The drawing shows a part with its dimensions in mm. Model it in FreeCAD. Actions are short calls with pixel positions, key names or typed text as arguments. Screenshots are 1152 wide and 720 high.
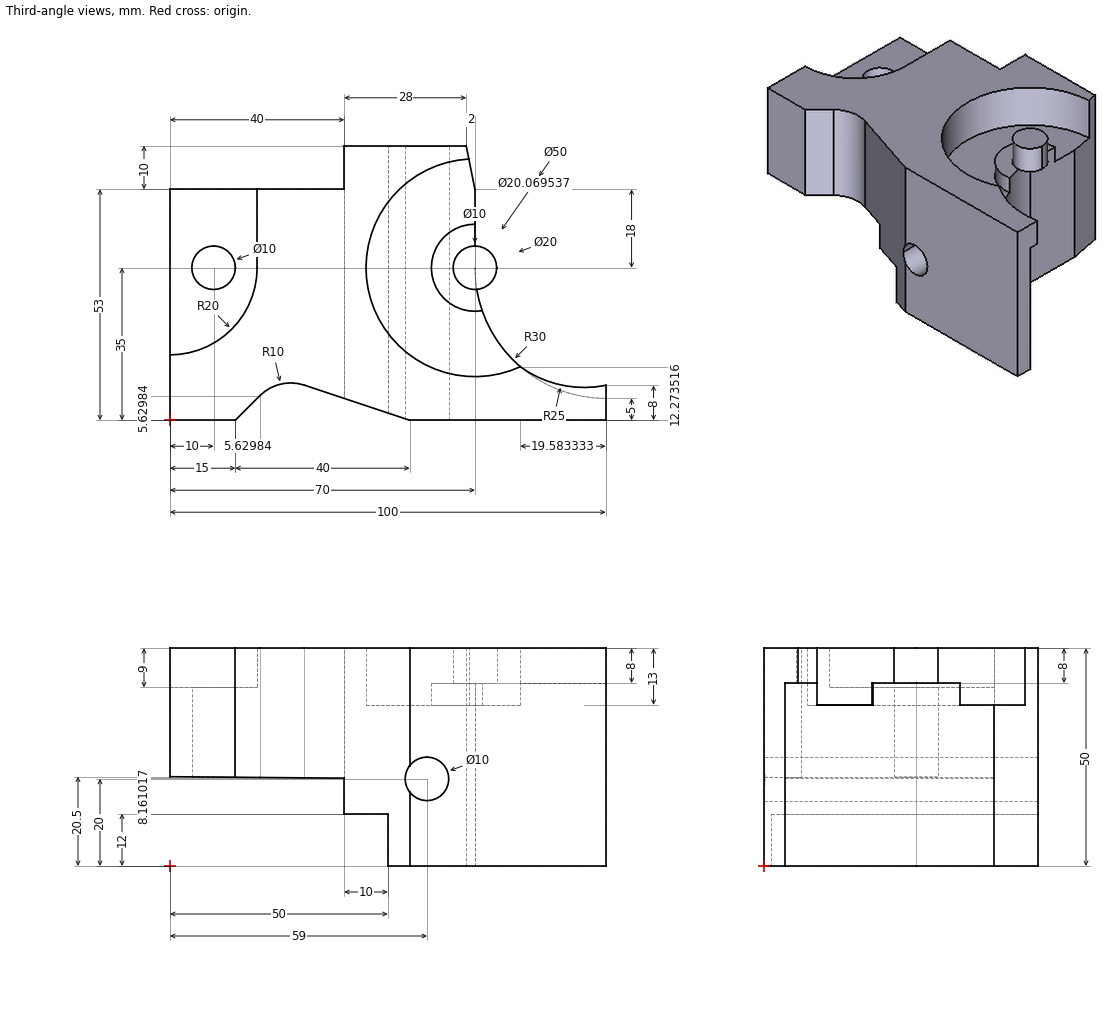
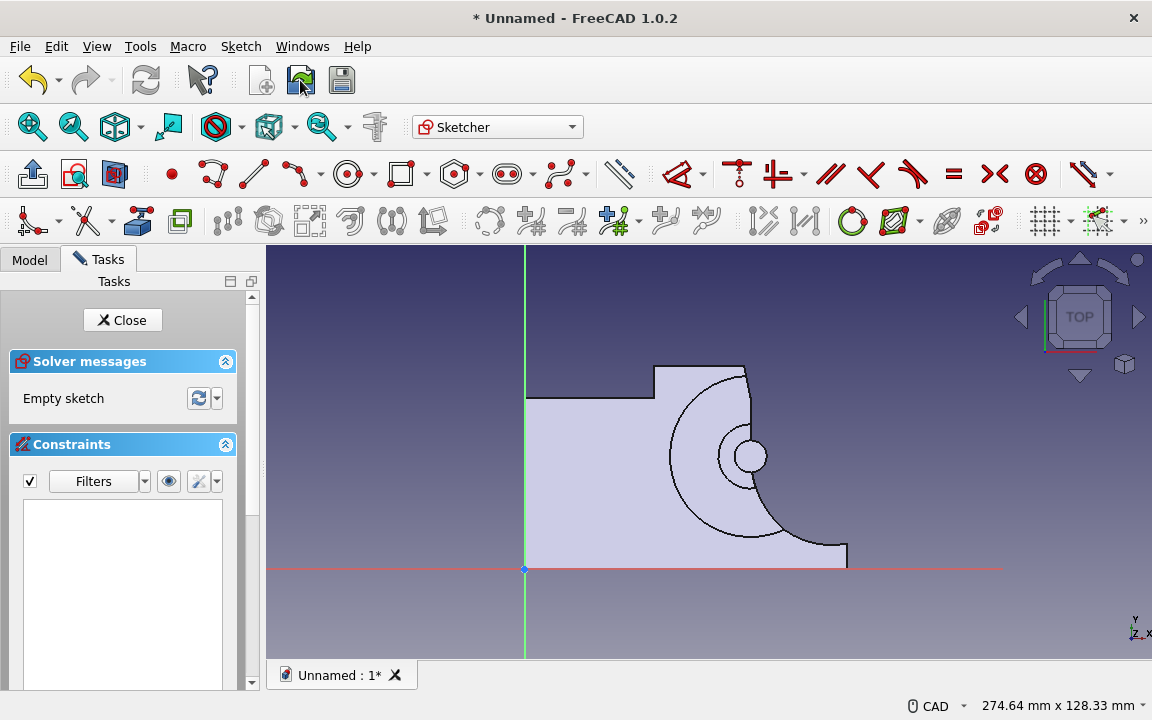
scroll(598, 616, up, 5)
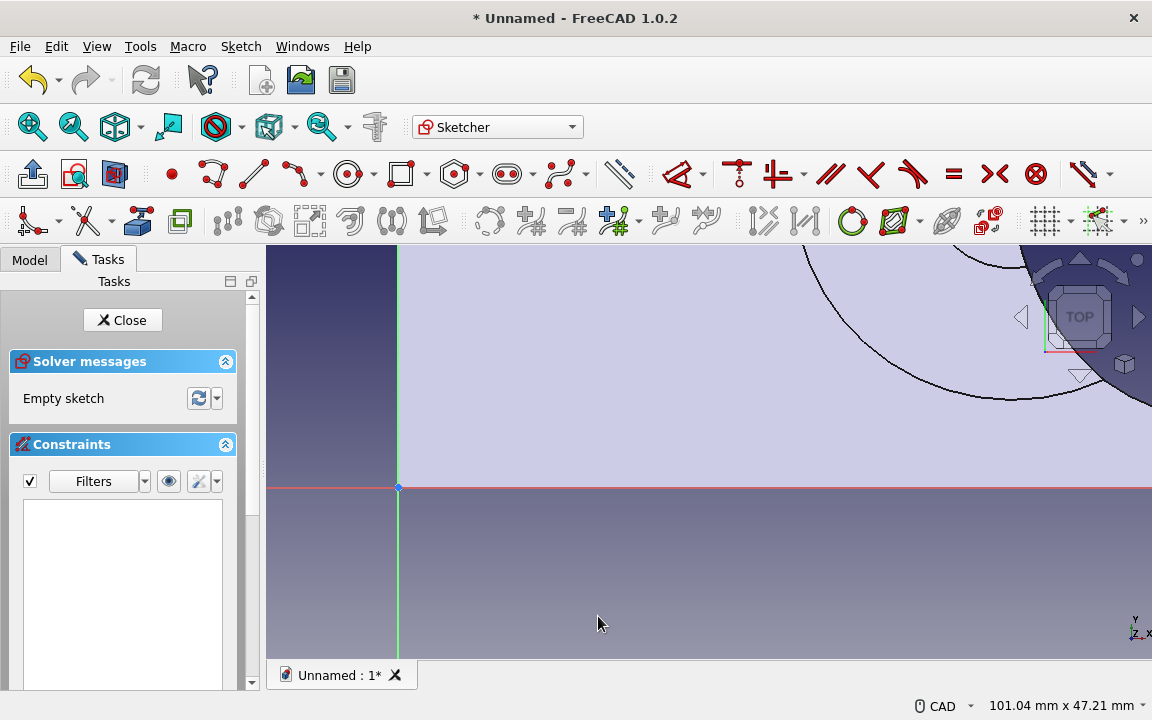
key(g)
key(m)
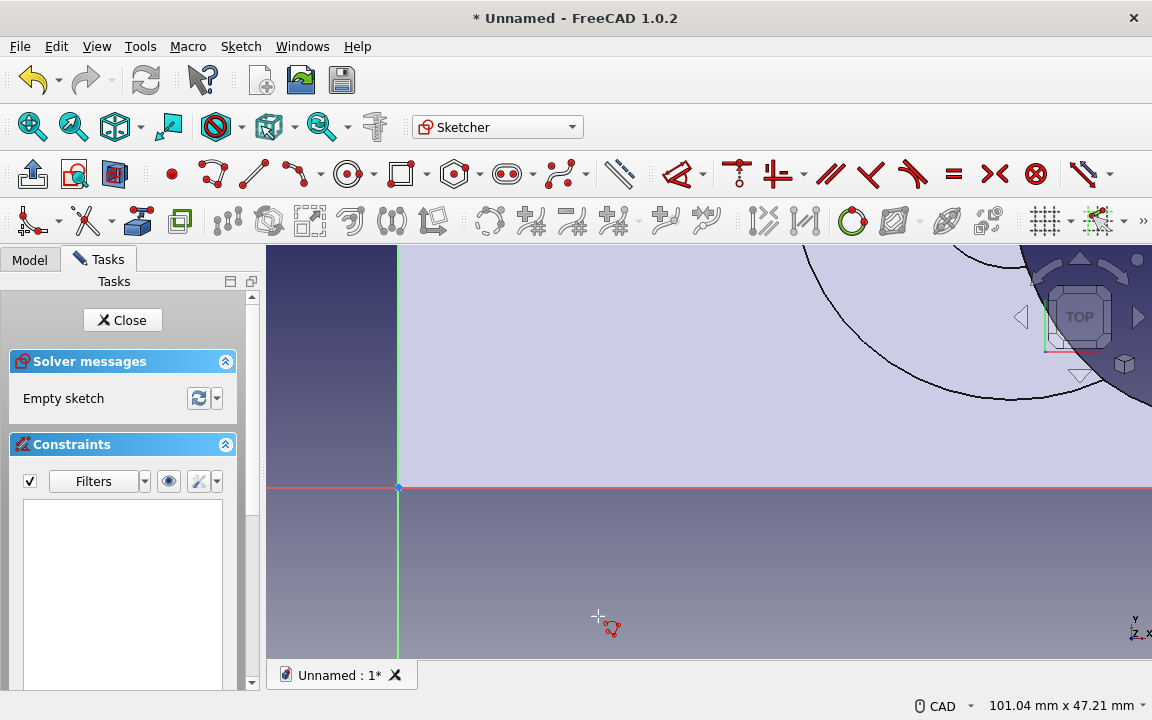
click(579, 438)
click(530, 488)
click(881, 479)
click(669, 417)
right_click(669, 417)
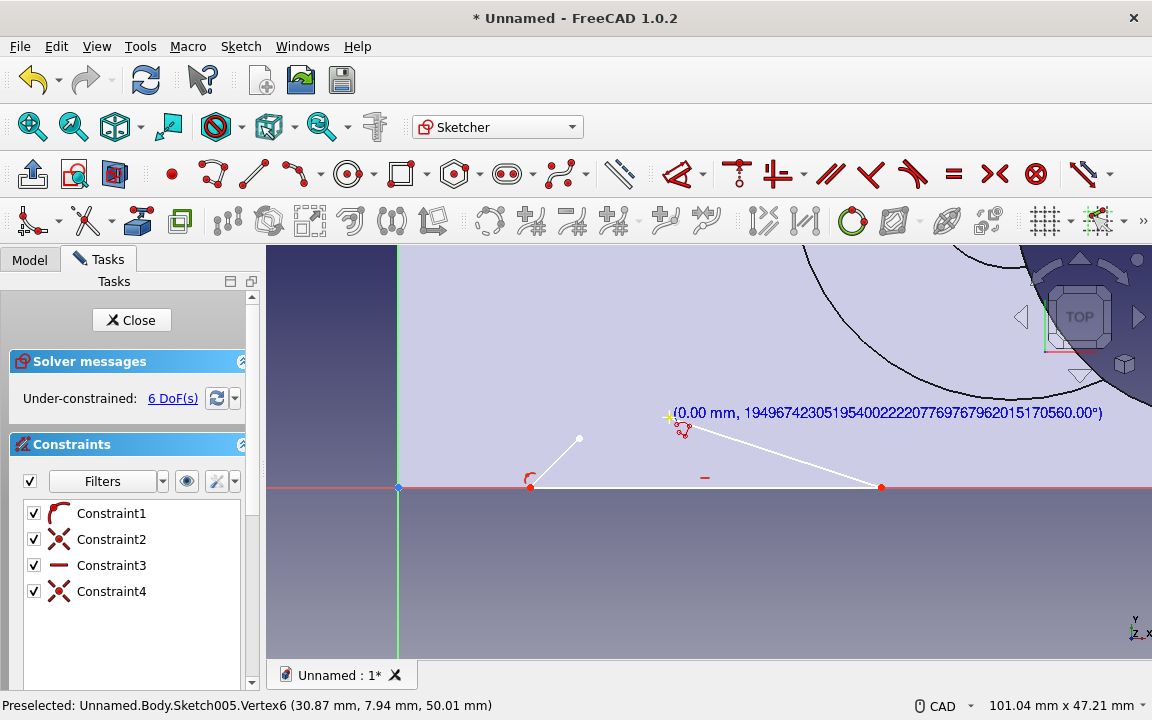
key(g)
key(3)
key(a)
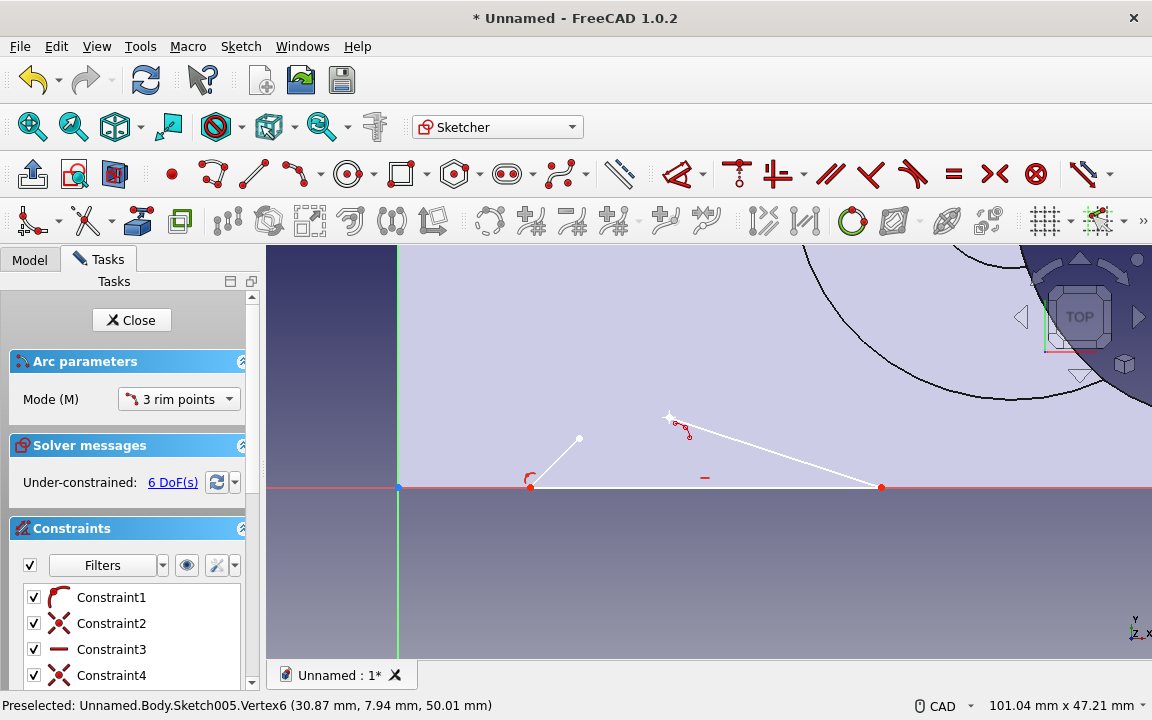
click(669, 418)
click(579, 439)
click(621, 415)
key(Escape)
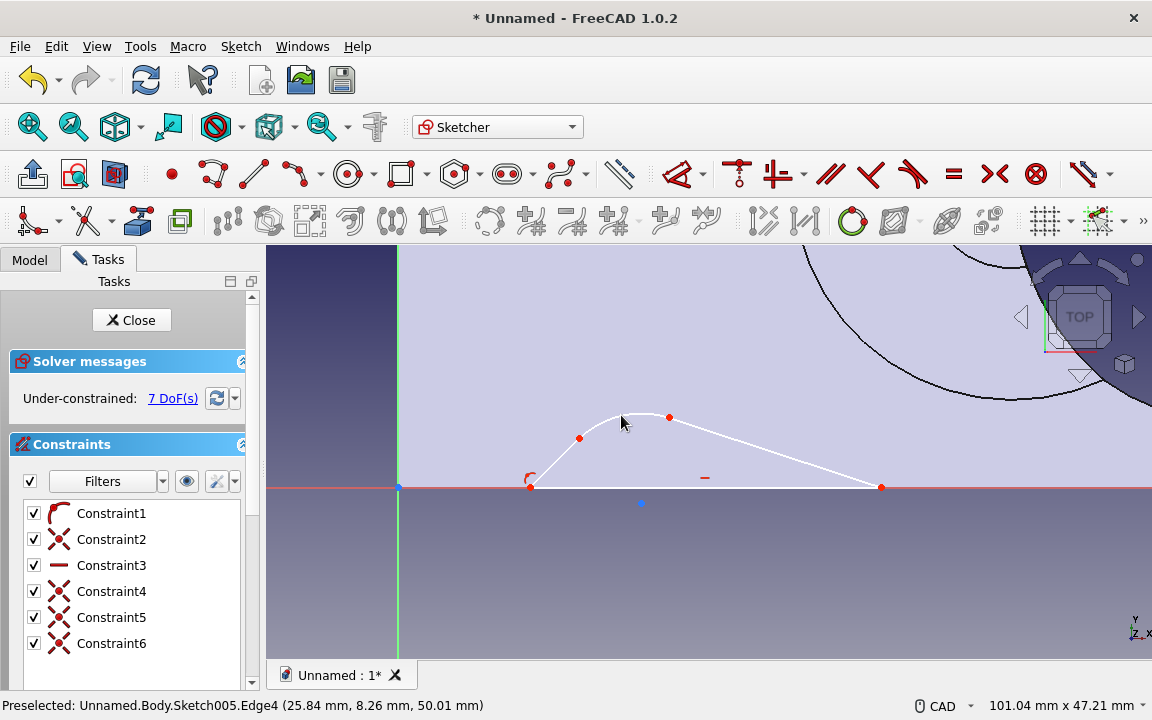
click(564, 454)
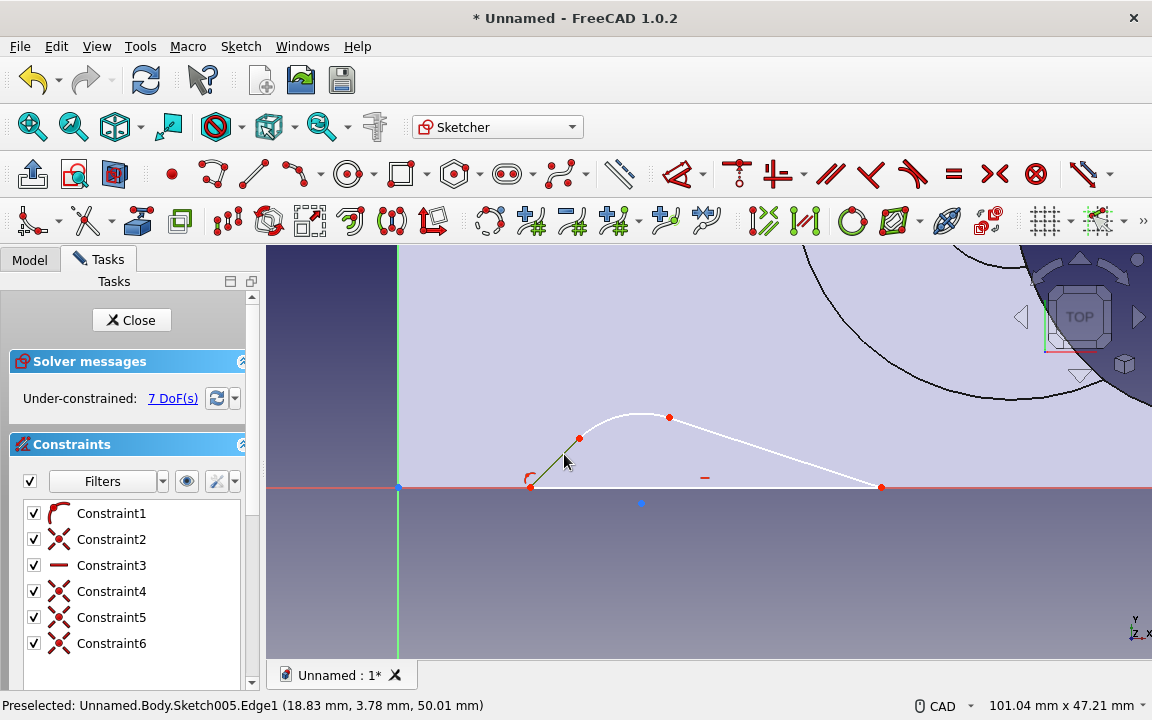
click(640, 414)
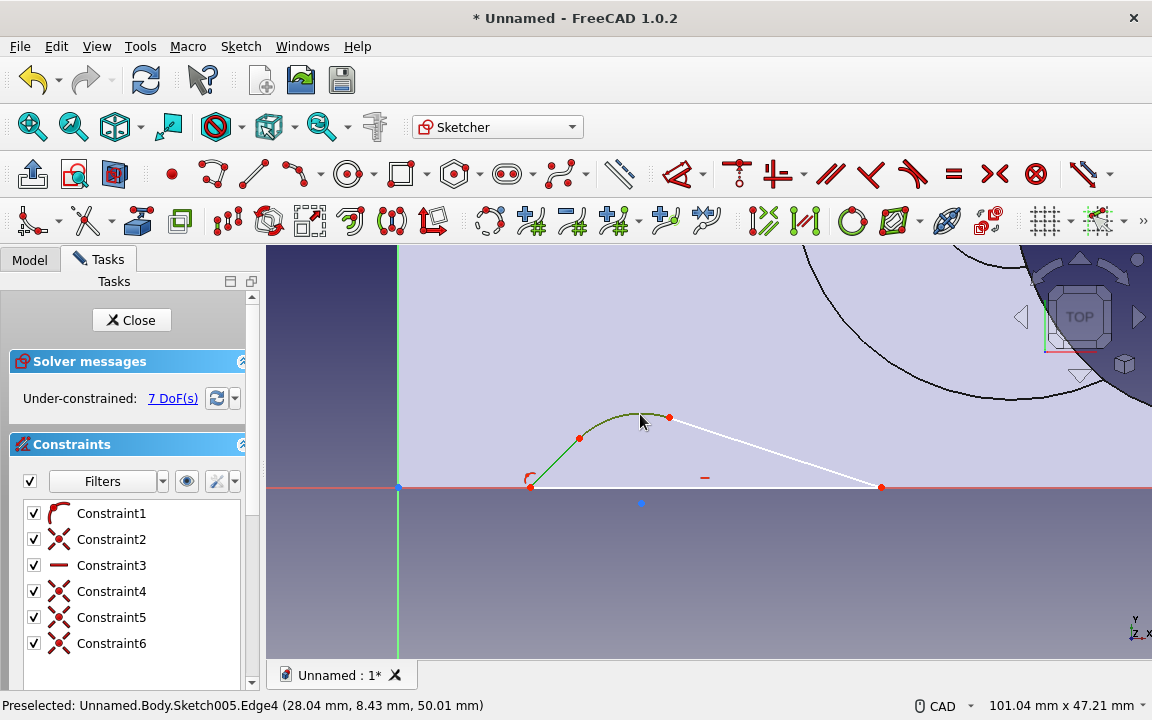
key(t)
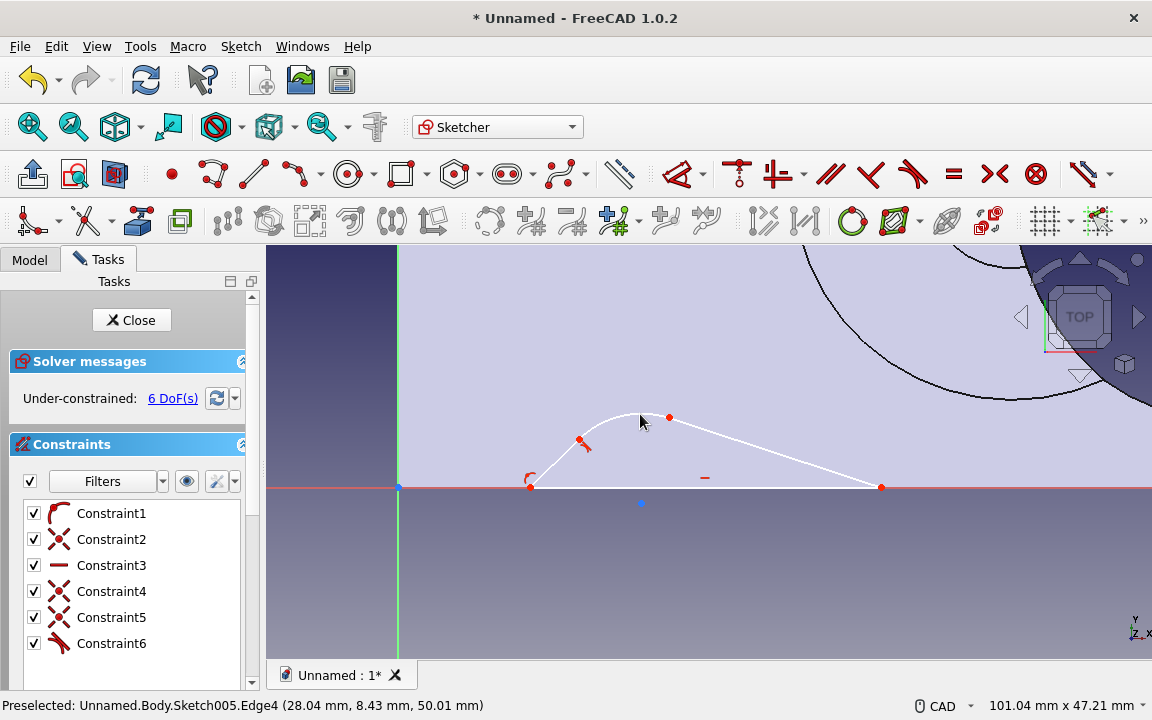
click(817, 467)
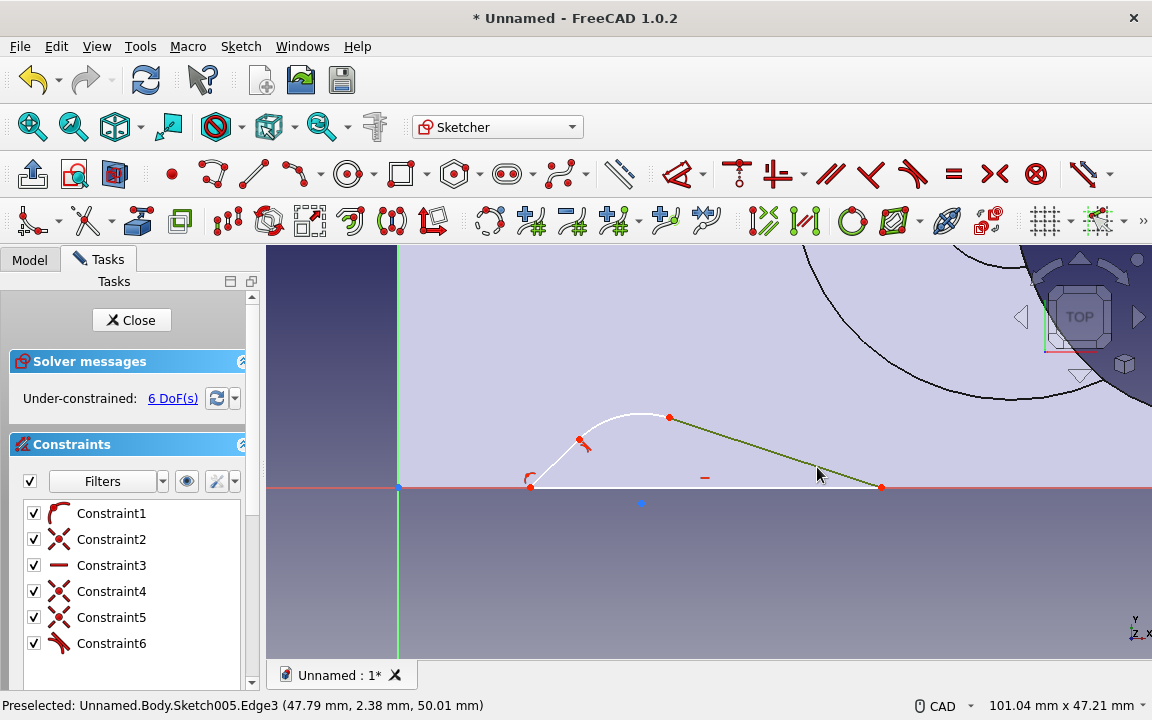
click(640, 414)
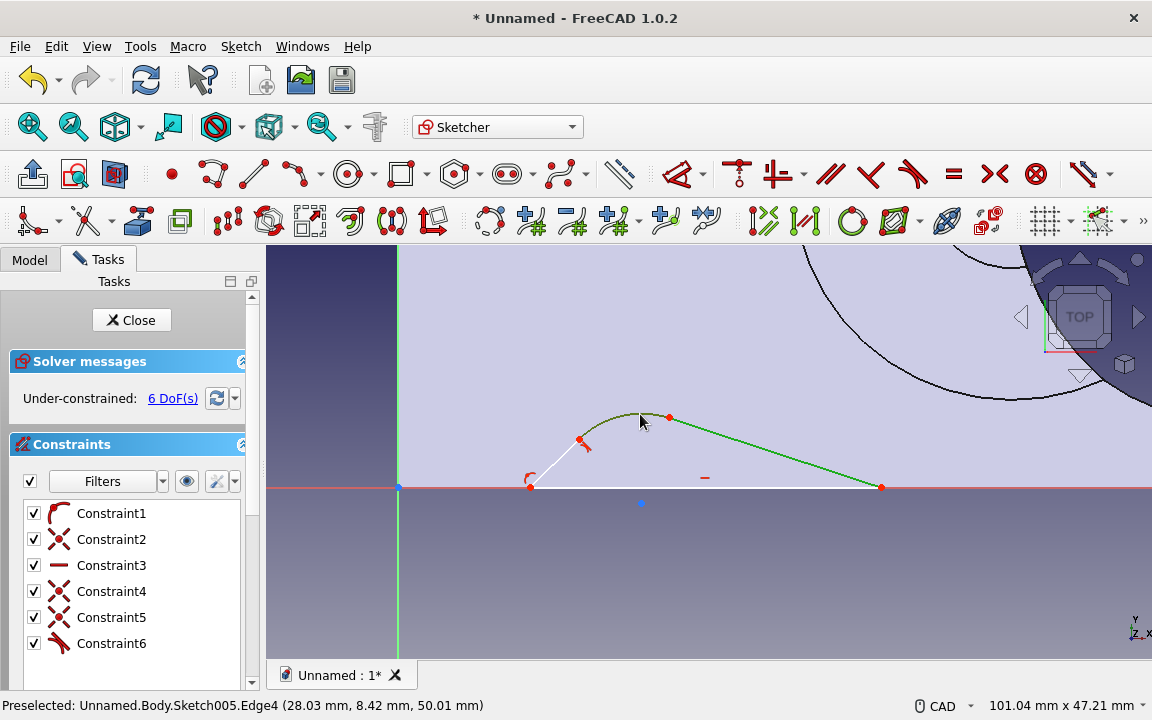
key(t)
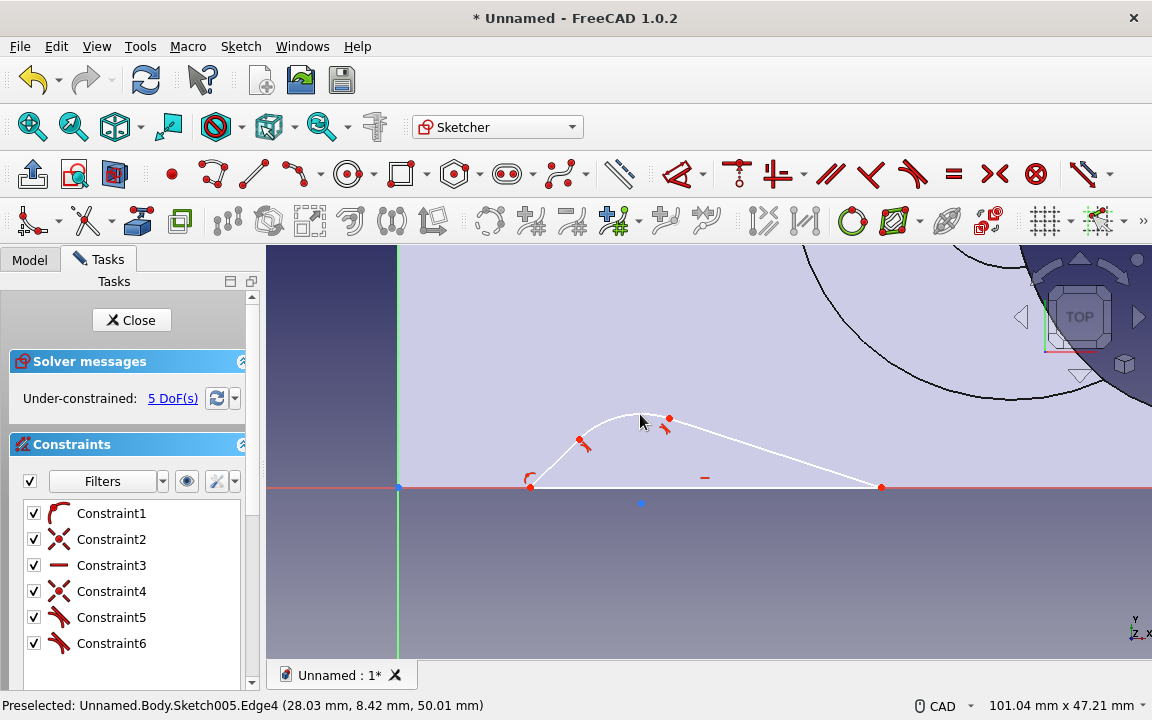
key(d)